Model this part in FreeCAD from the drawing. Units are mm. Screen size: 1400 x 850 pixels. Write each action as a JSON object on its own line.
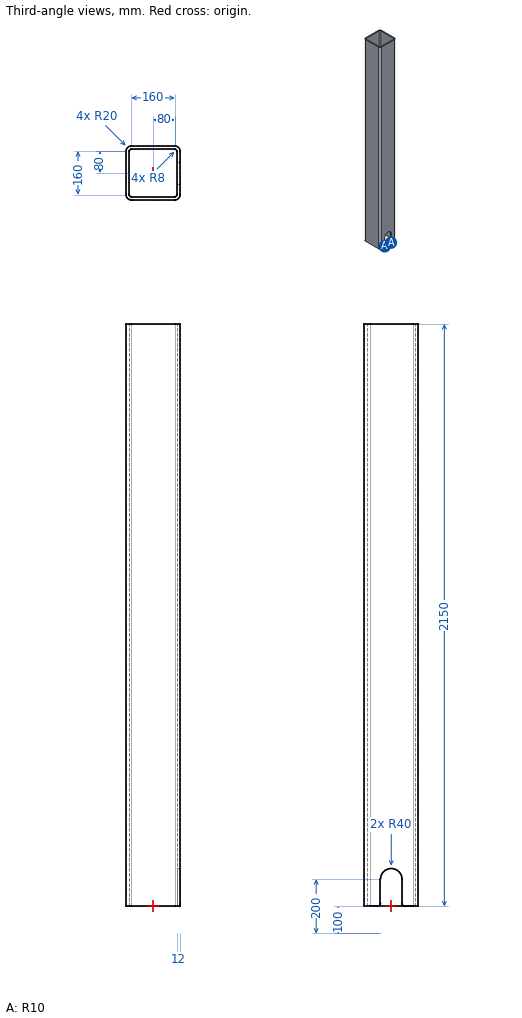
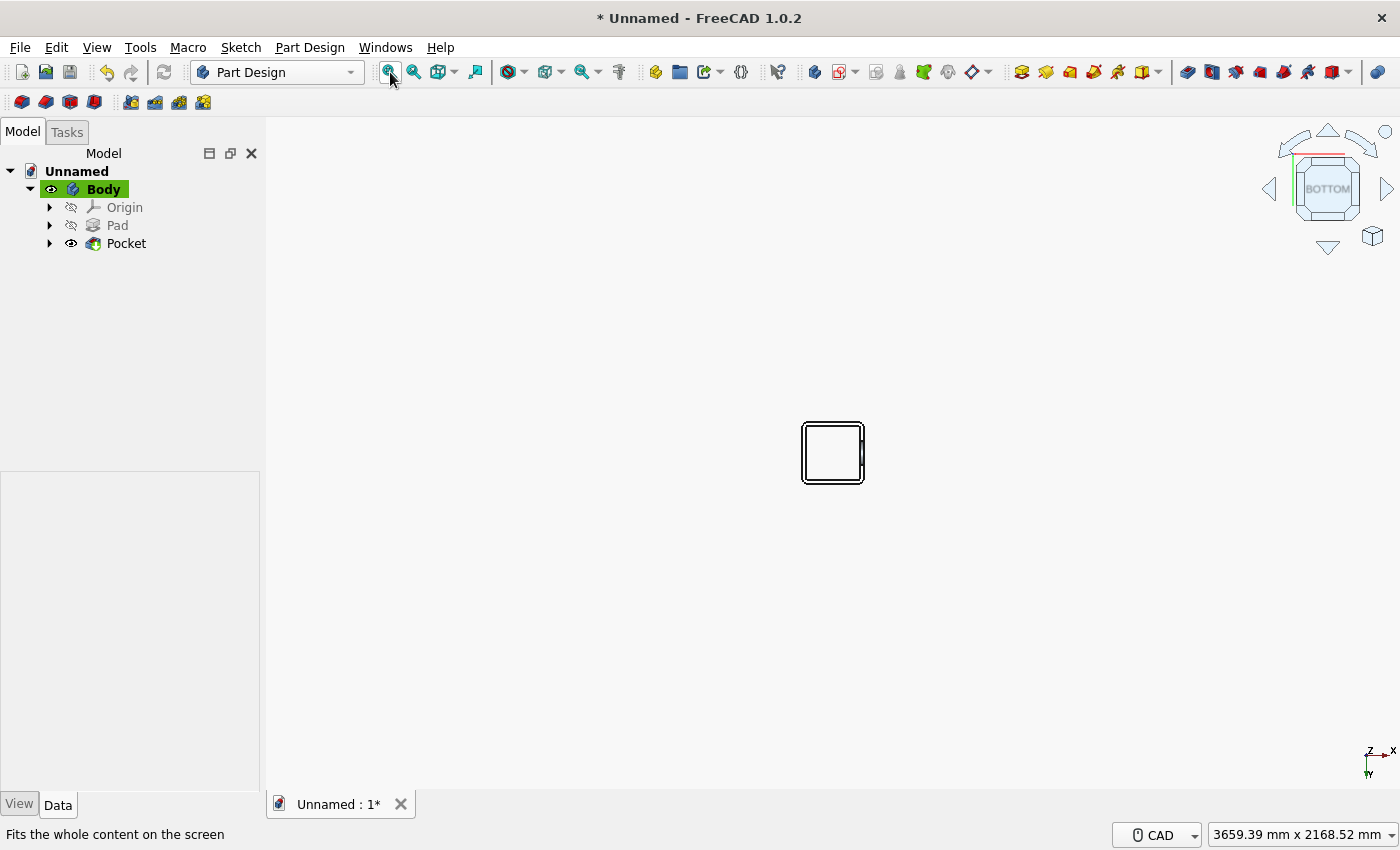
{"action": "scroll", "coordinate": [862, 440], "scroll_direction": "up", "scroll_amount": 12}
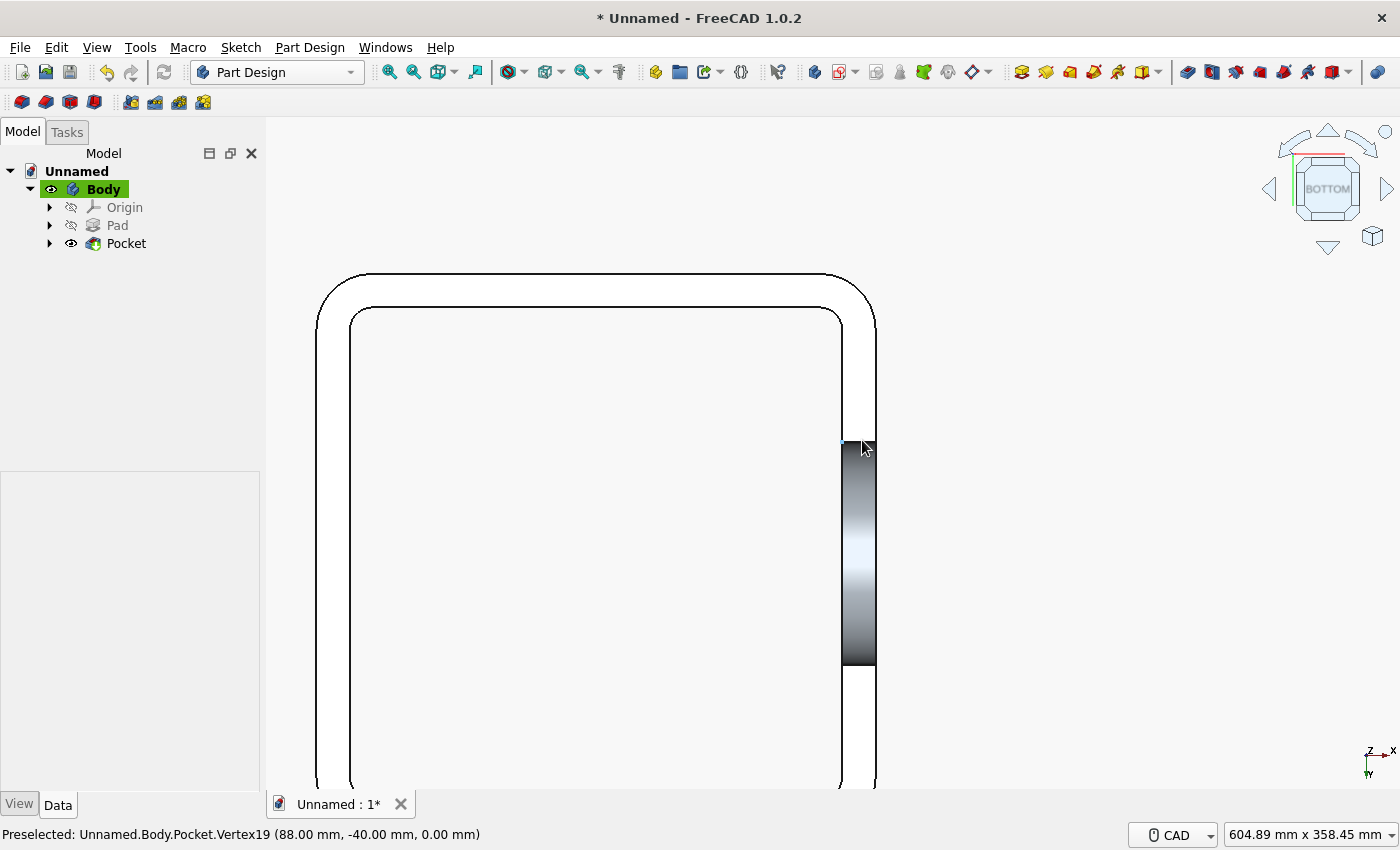
{"action": "left_click", "coordinate": [858, 441]}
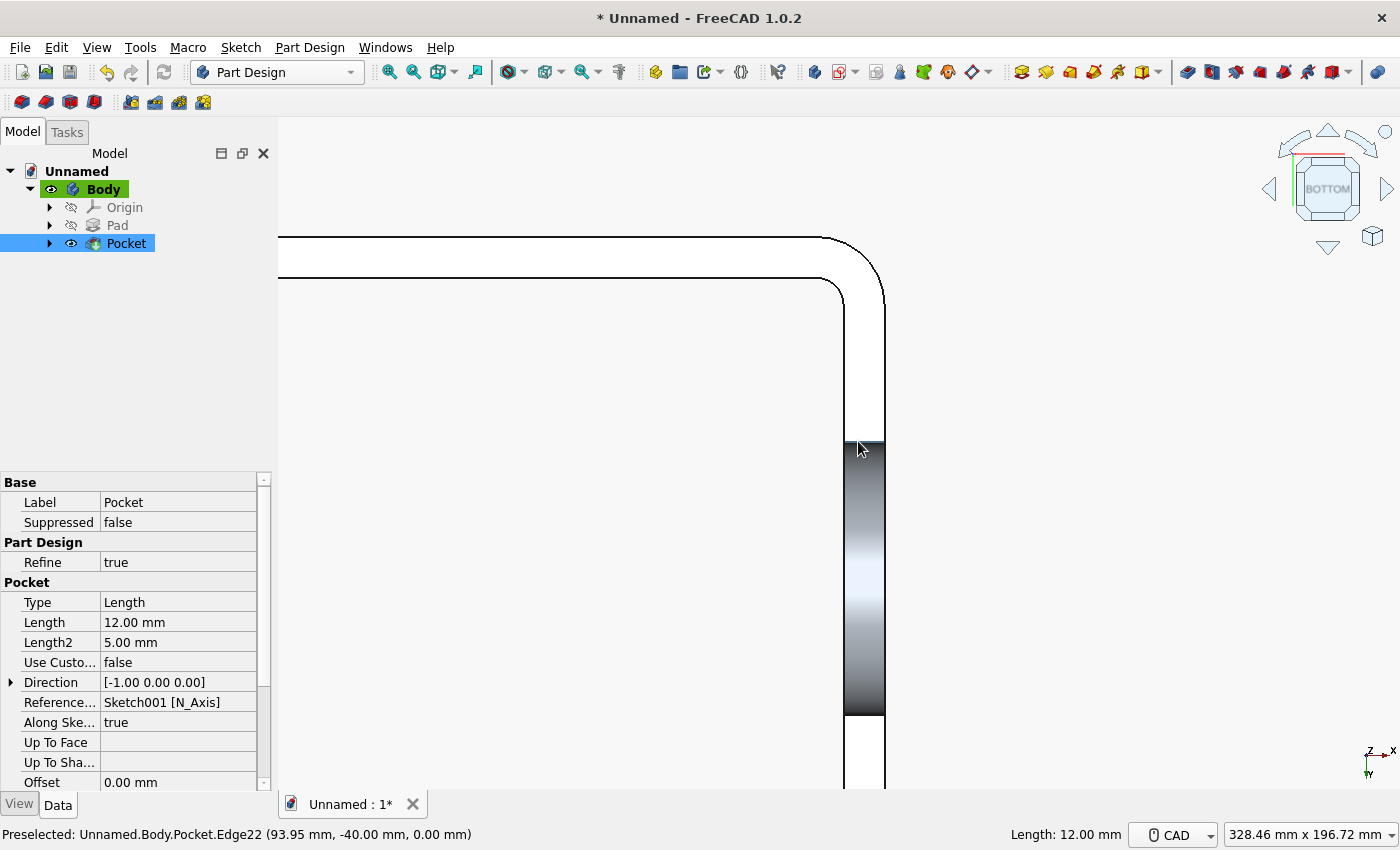
{"action": "left_click", "coordinate": [864, 714], "text": "ctrl"}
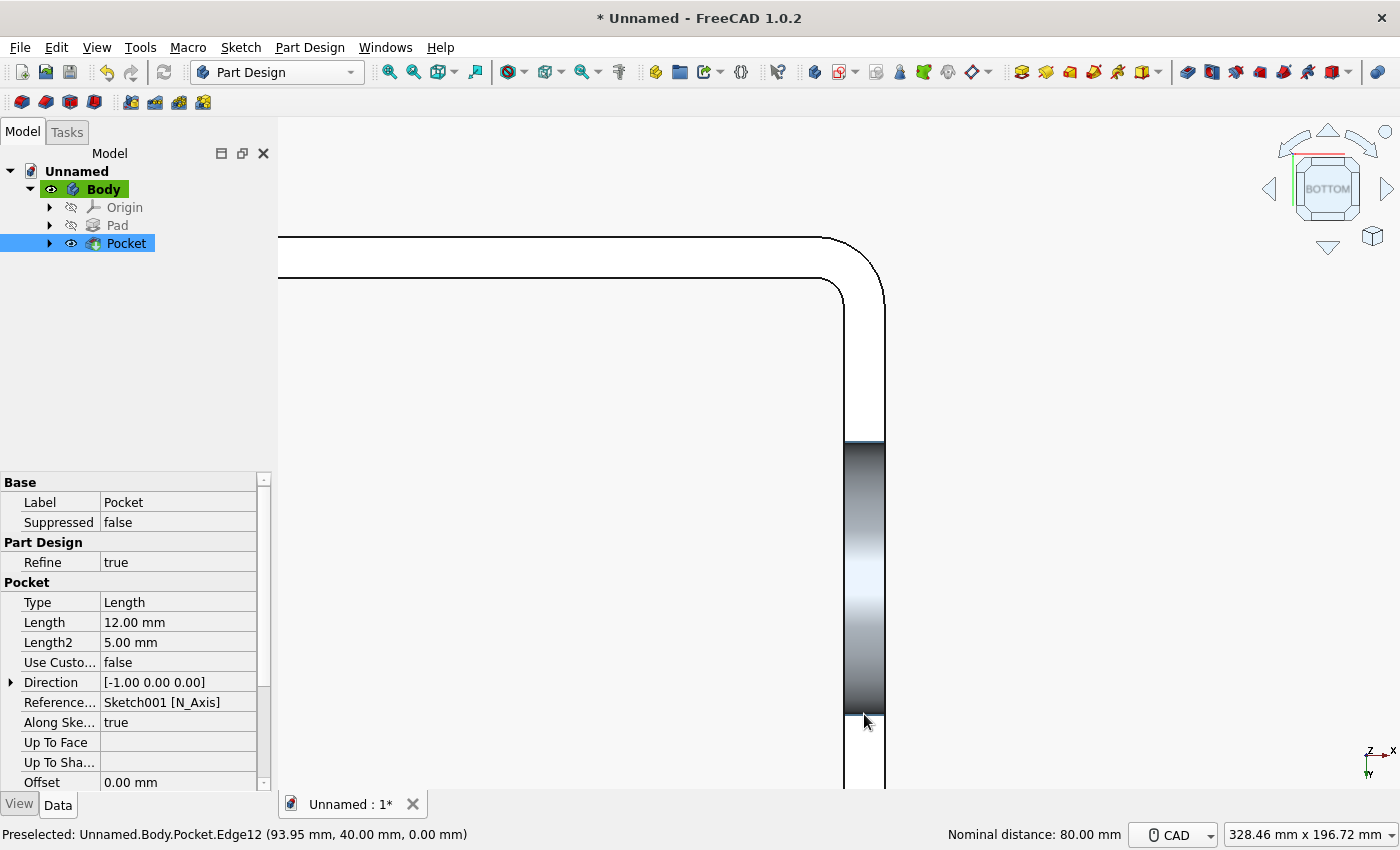
{"action": "left_click", "coordinate": [22, 102]}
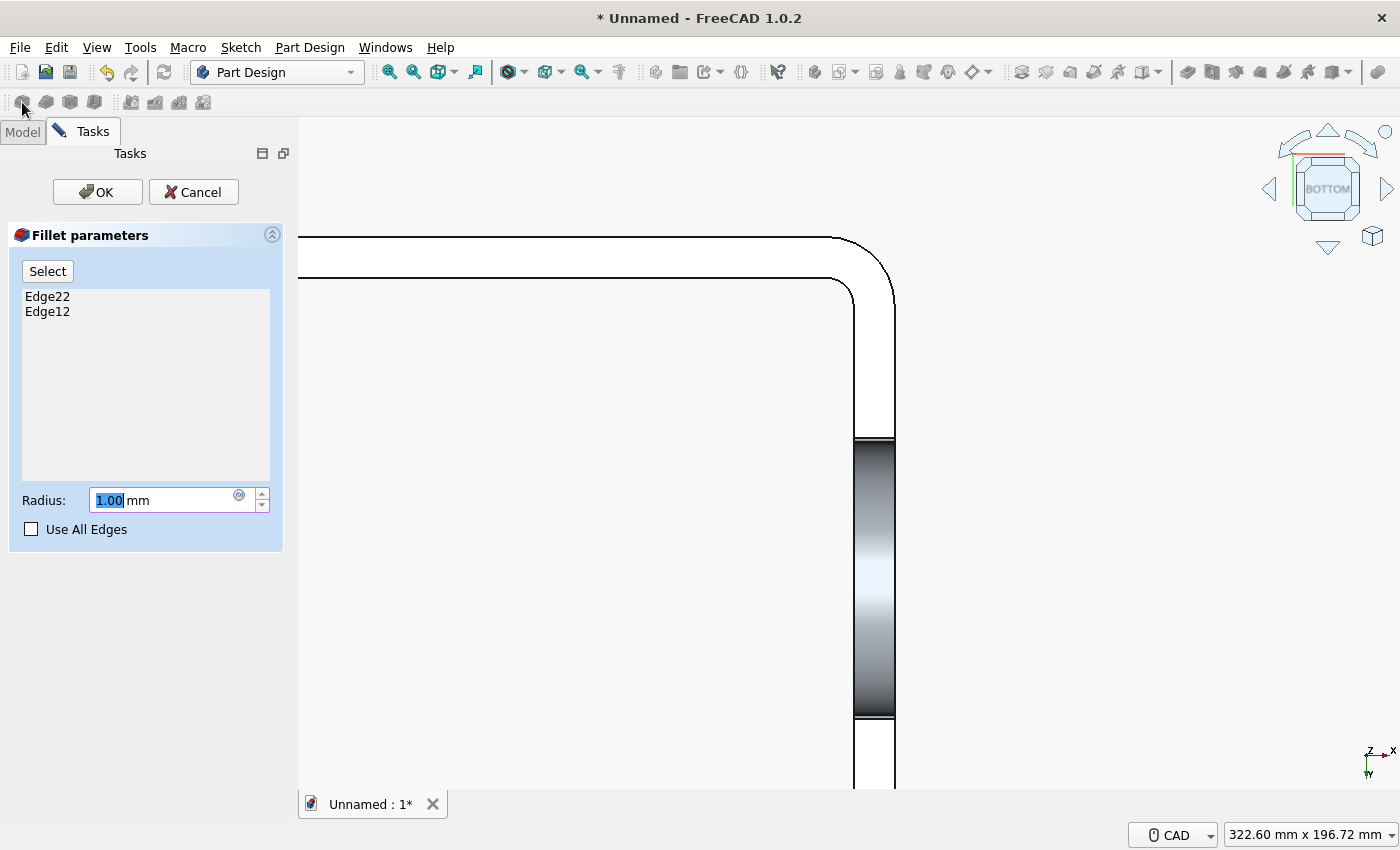
{"action": "type", "text": "10"}
{"action": "key", "text": "Tab"}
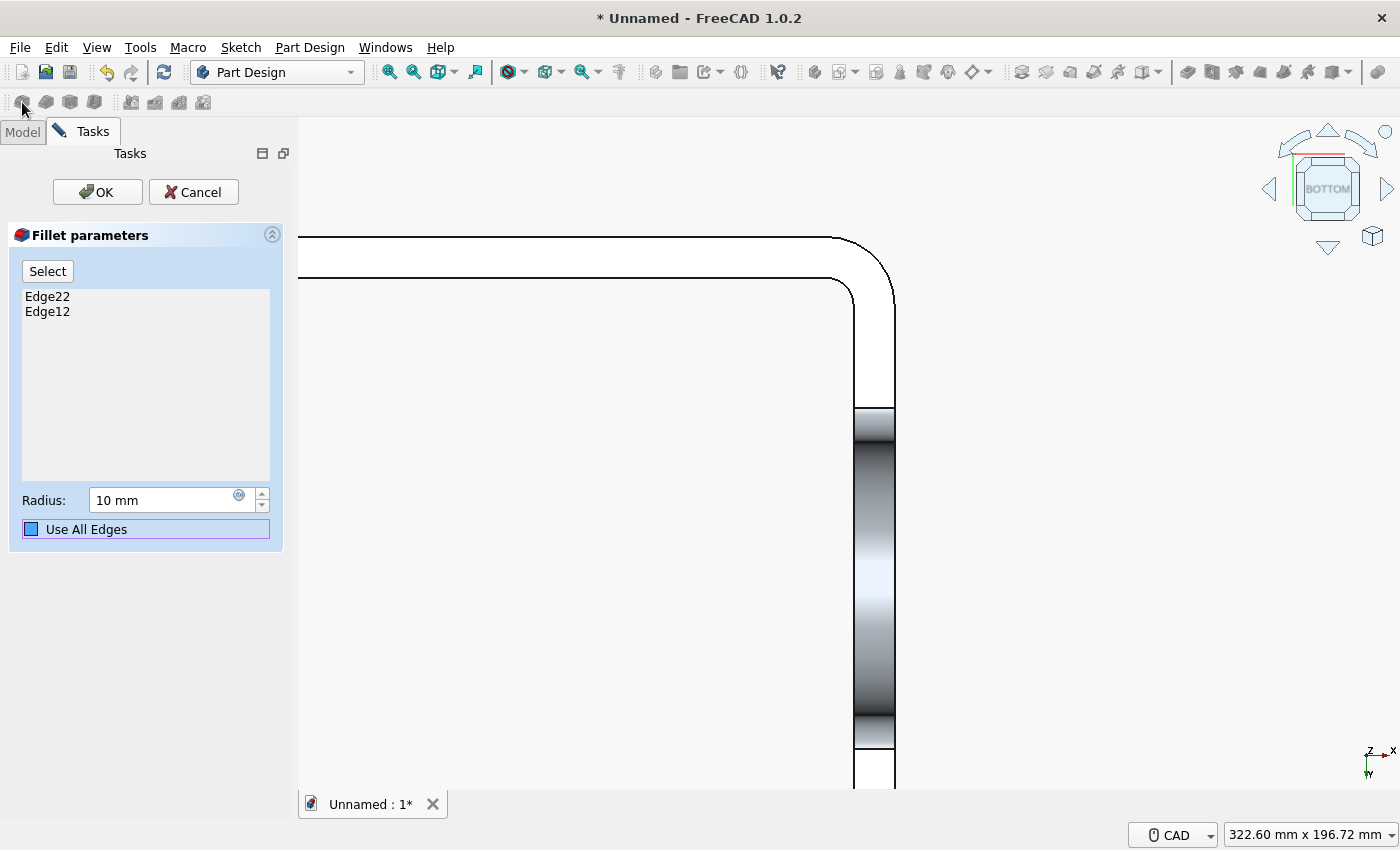
{"action": "left_click", "coordinate": [98, 192]}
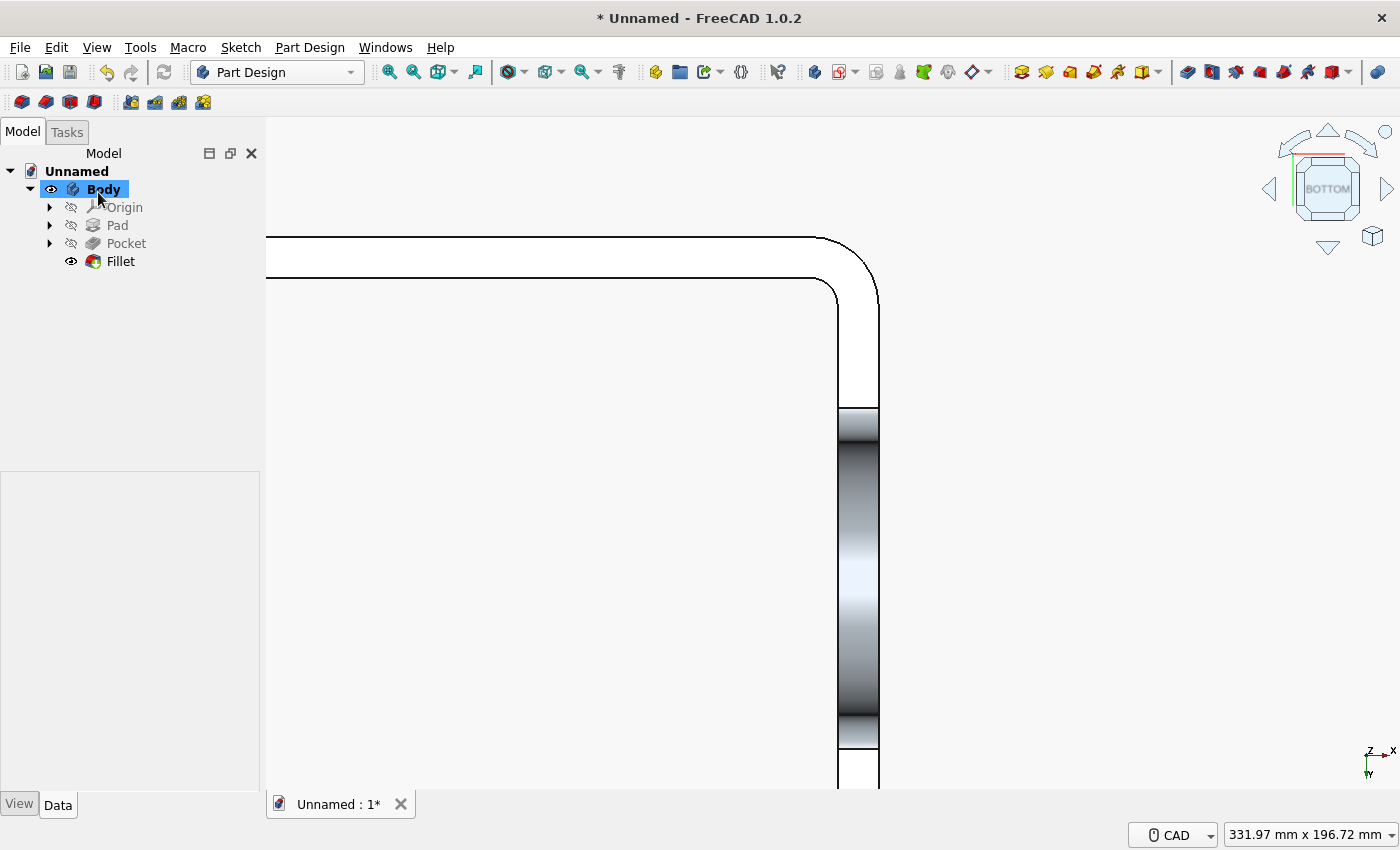
{"action": "key", "text": "0"}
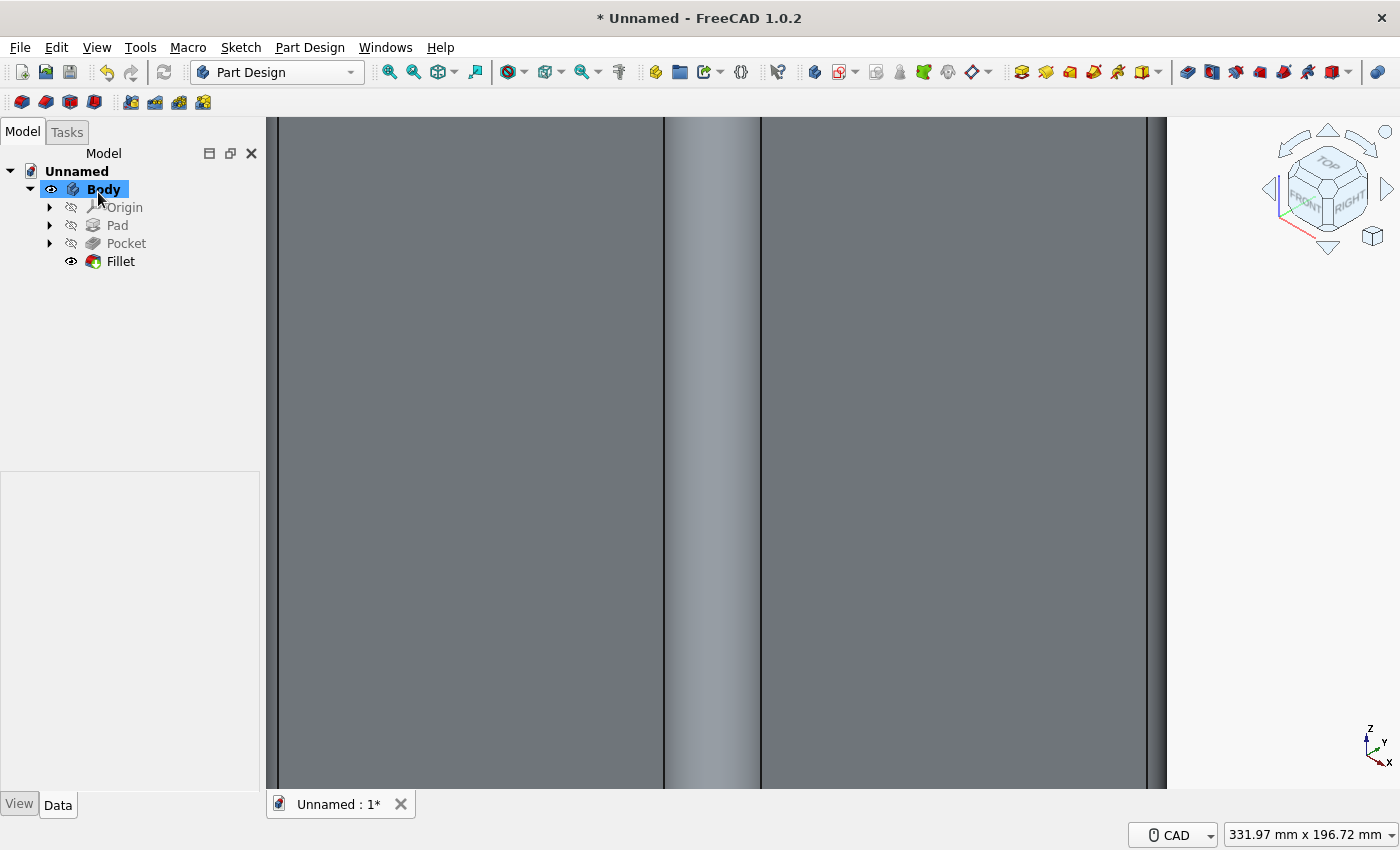
{"action": "left_click", "coordinate": [390, 72]}